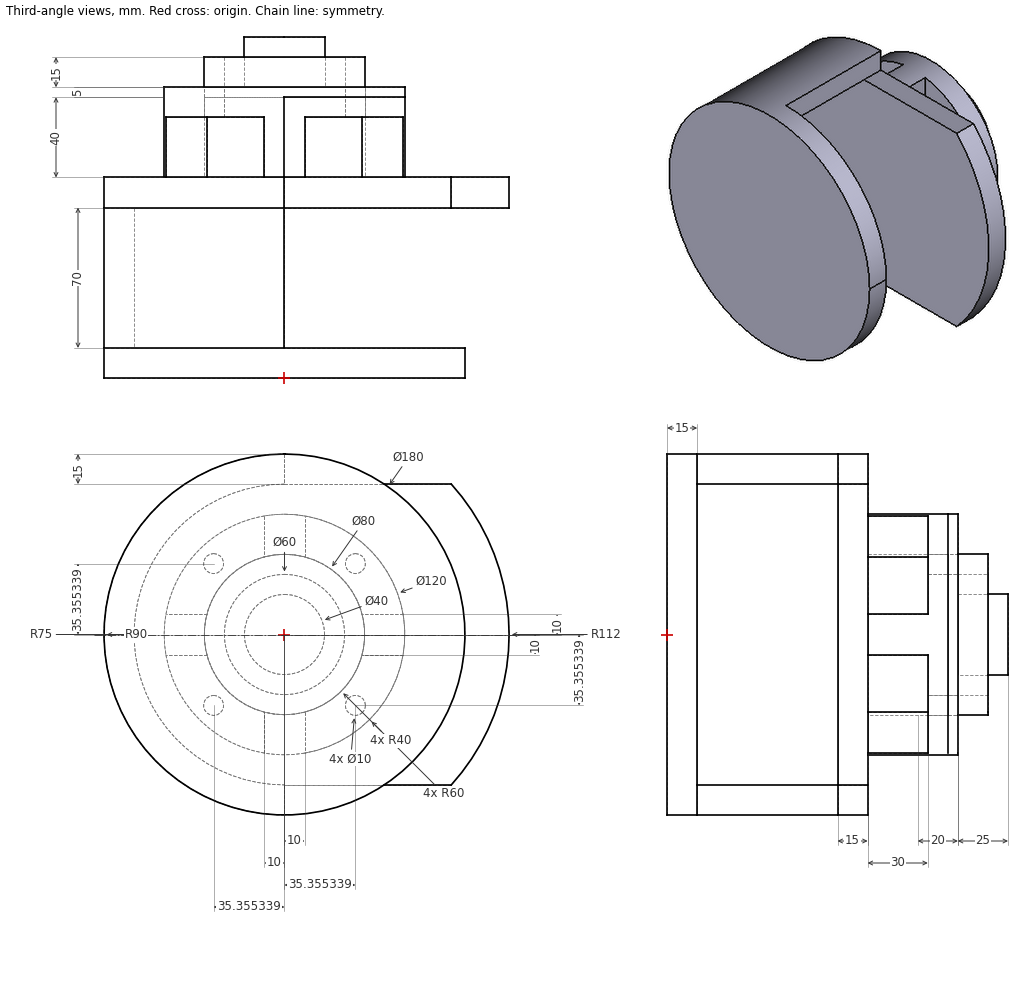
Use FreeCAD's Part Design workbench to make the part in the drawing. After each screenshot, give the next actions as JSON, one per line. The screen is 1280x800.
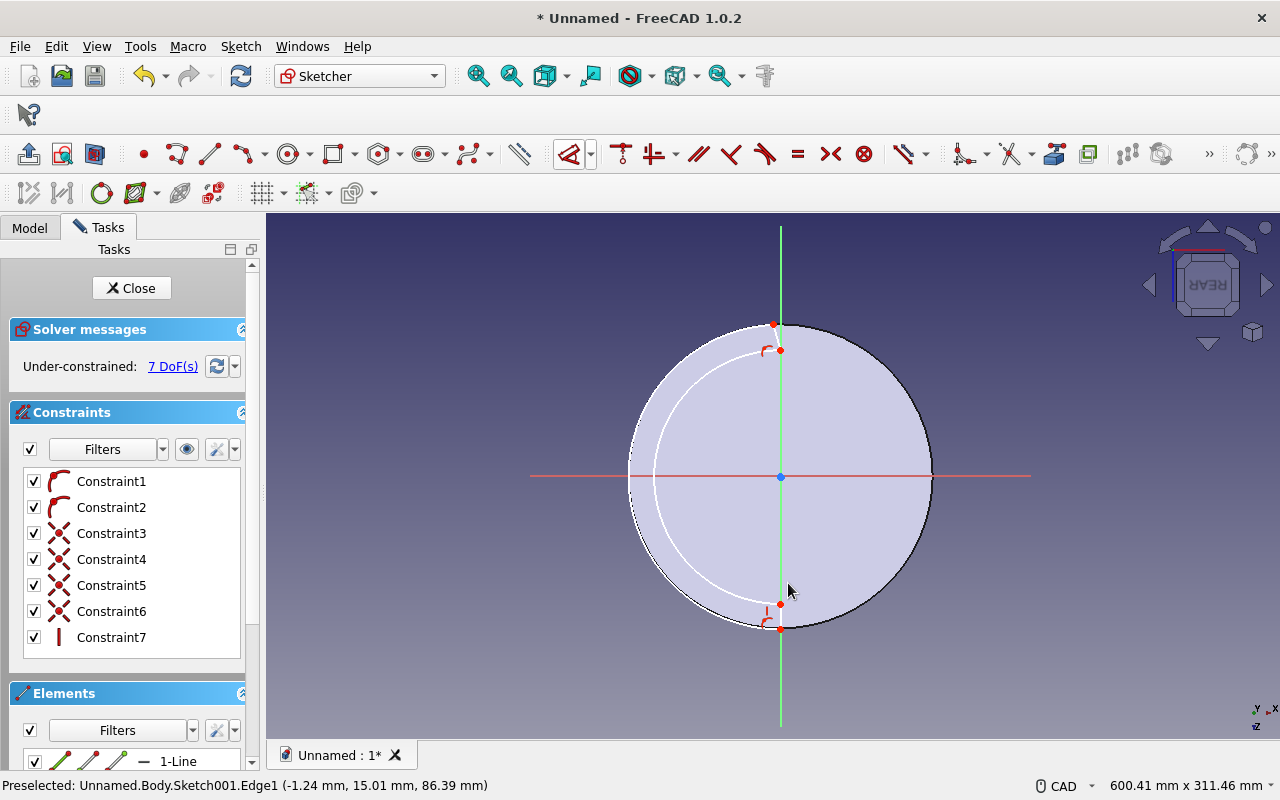
{"action": "scroll", "coordinate": [776, 332], "scroll_direction": "up", "scroll_amount": 5}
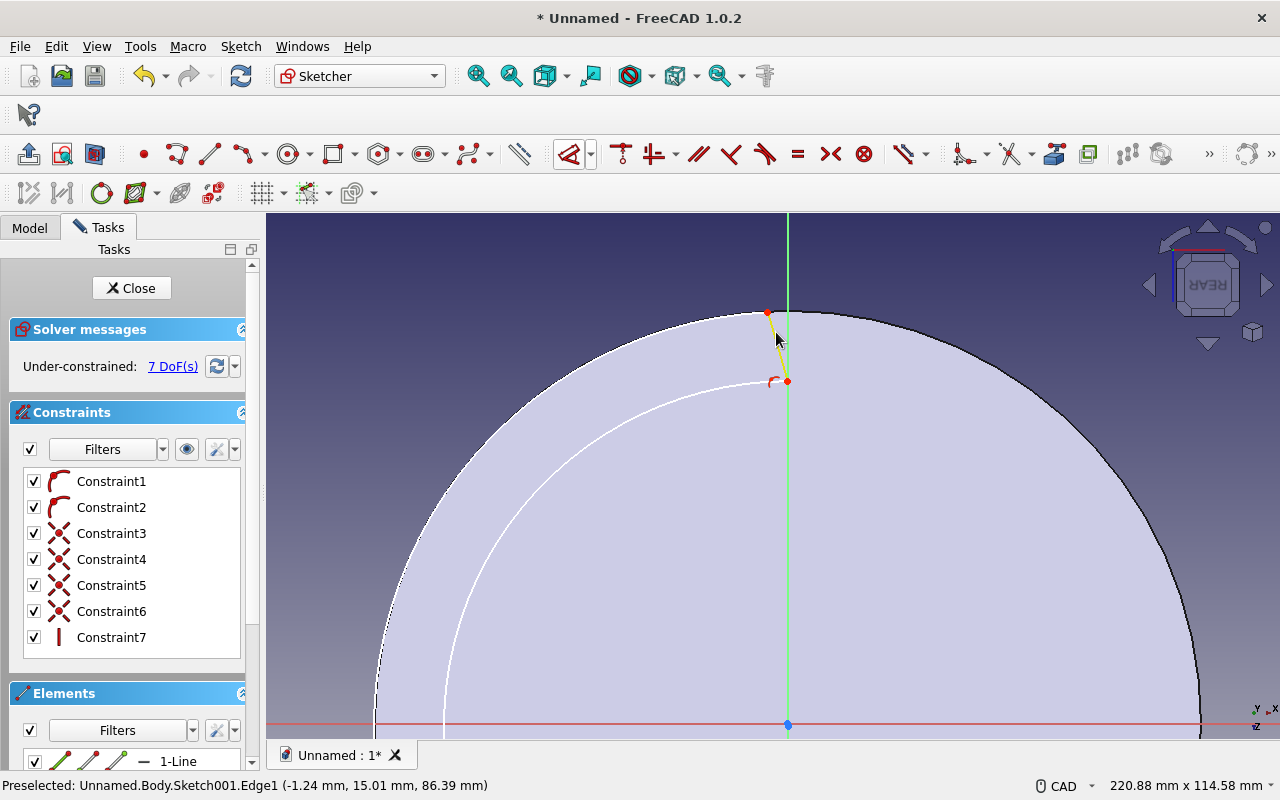
{"action": "left_click", "coordinate": [774, 333]}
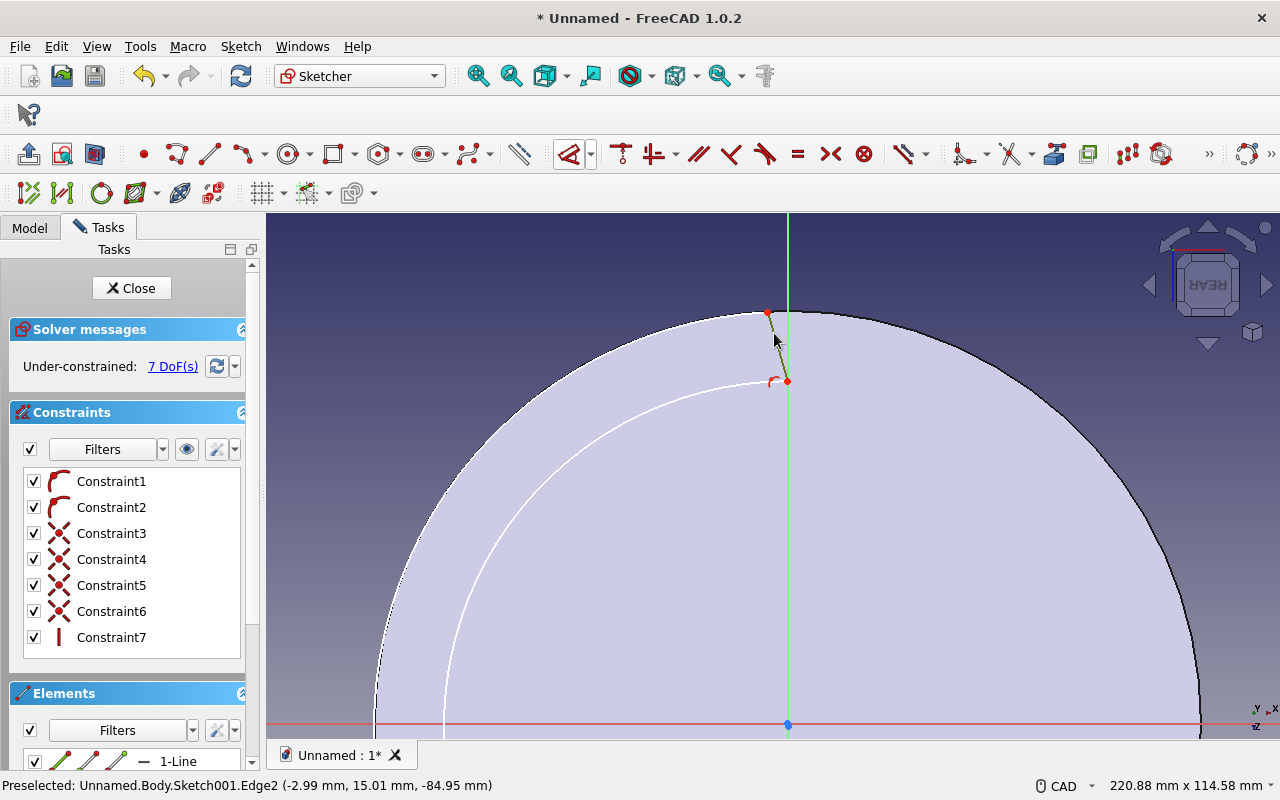
{"action": "key", "text": "v"}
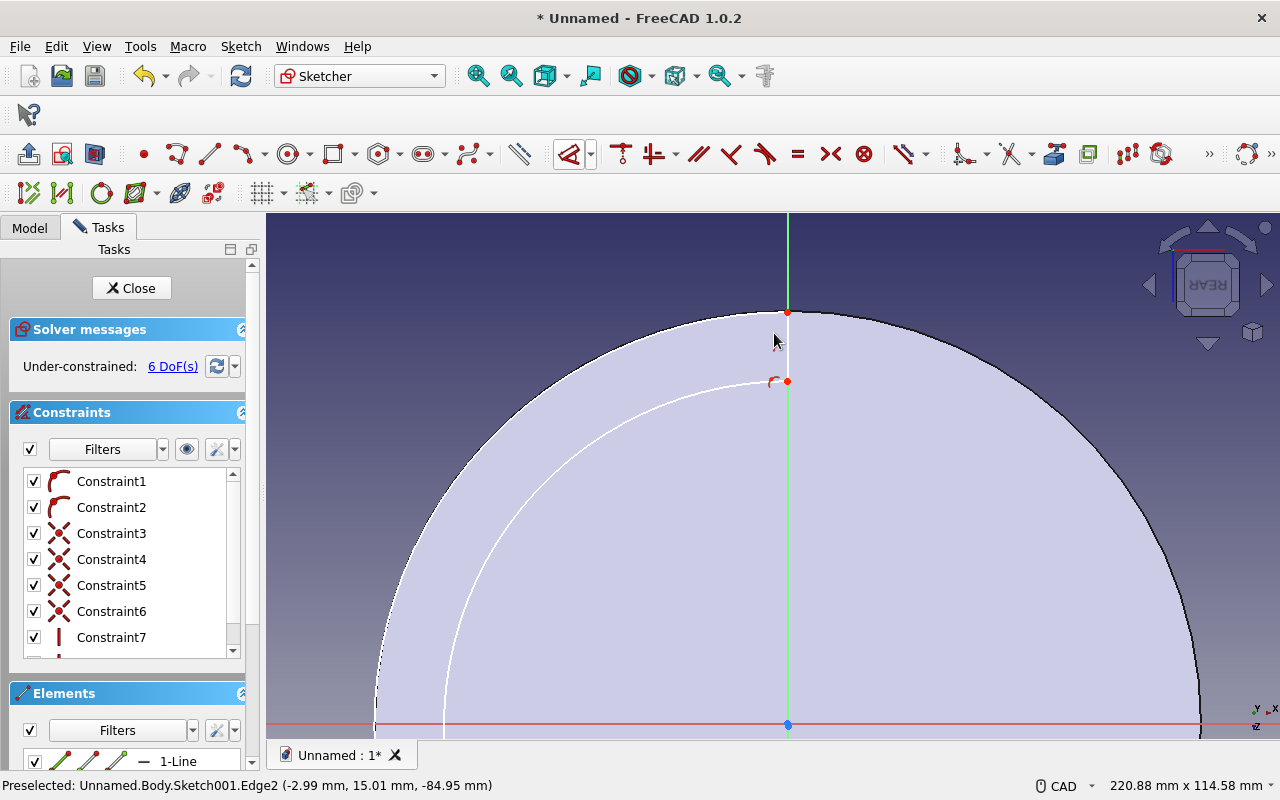
{"action": "left_click", "coordinate": [510, 524]}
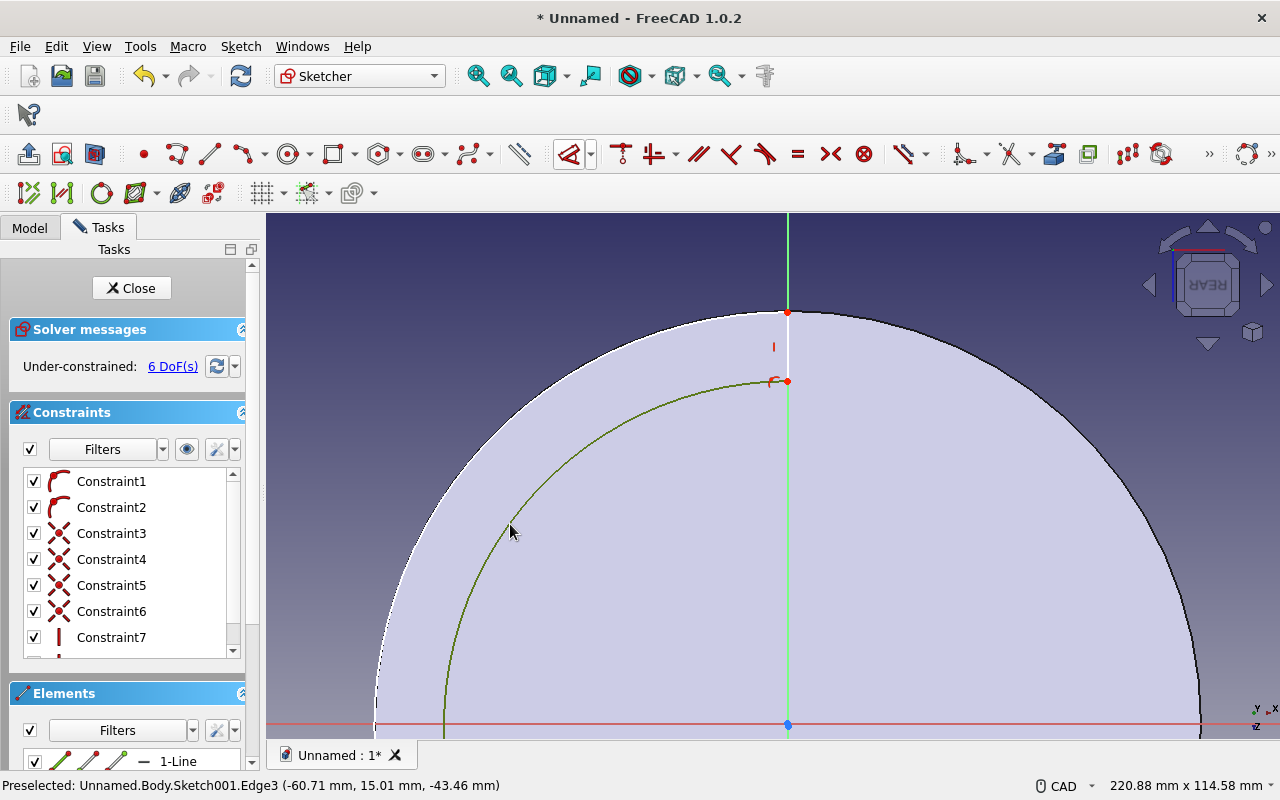
{"action": "left_click", "coordinate": [453, 483]}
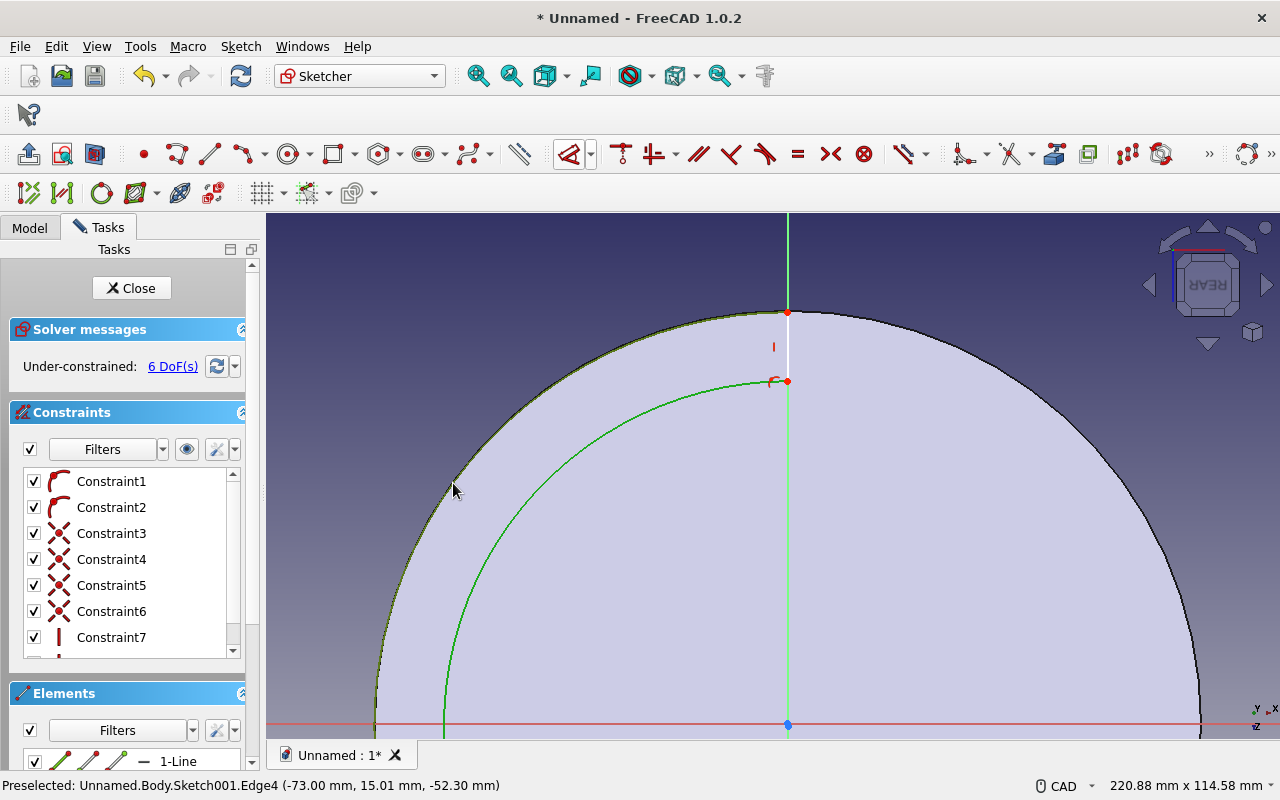
{"action": "left_click", "coordinate": [621, 154]}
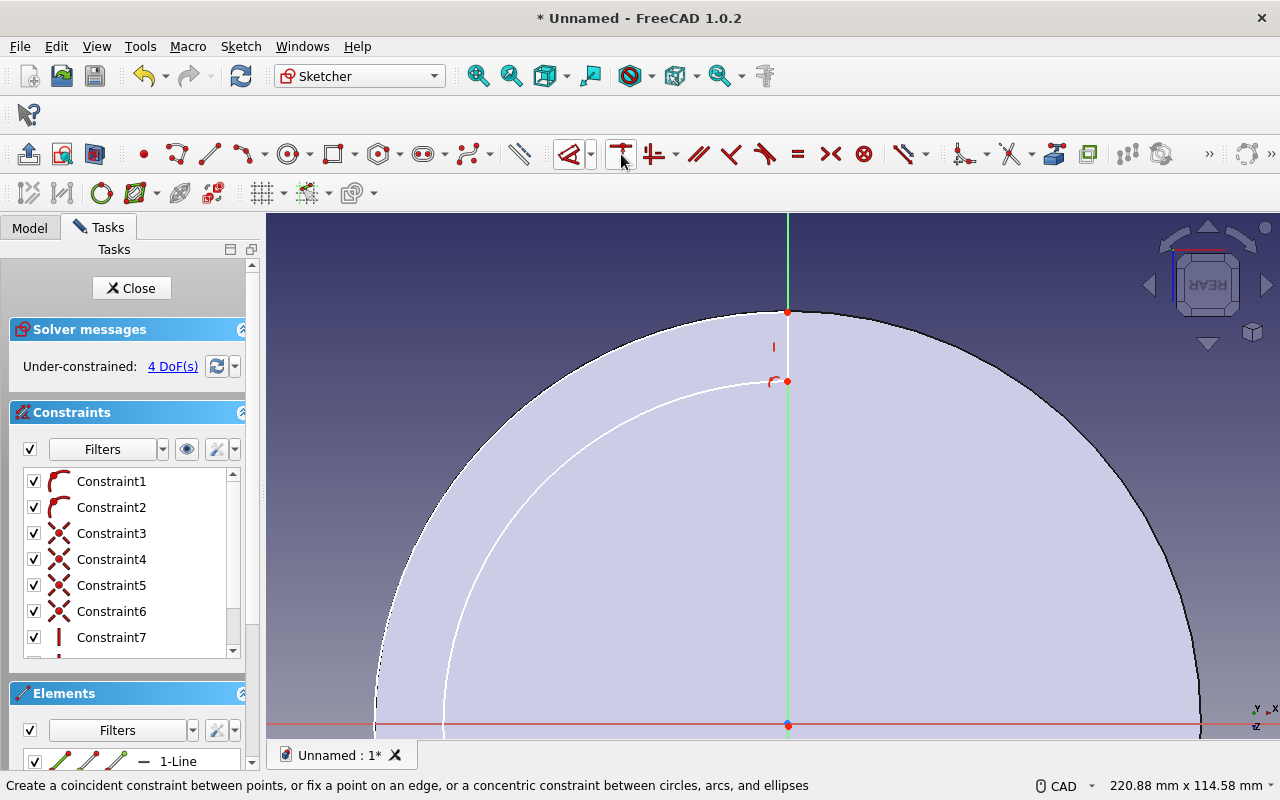
{"action": "scroll", "coordinate": [776, 332], "scroll_direction": "down", "scroll_amount": 5}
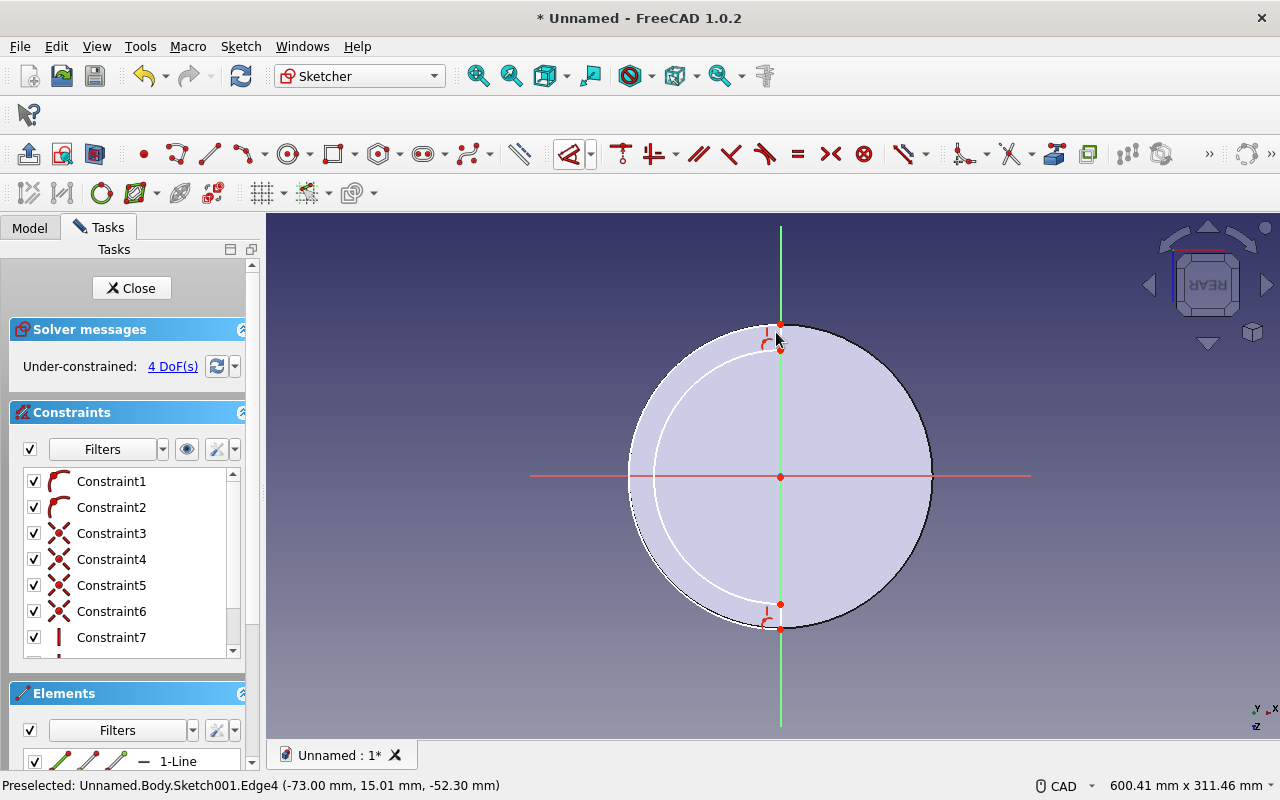
{"action": "left_click_drag", "start_coordinate": [771, 466], "coordinate": [791, 487]}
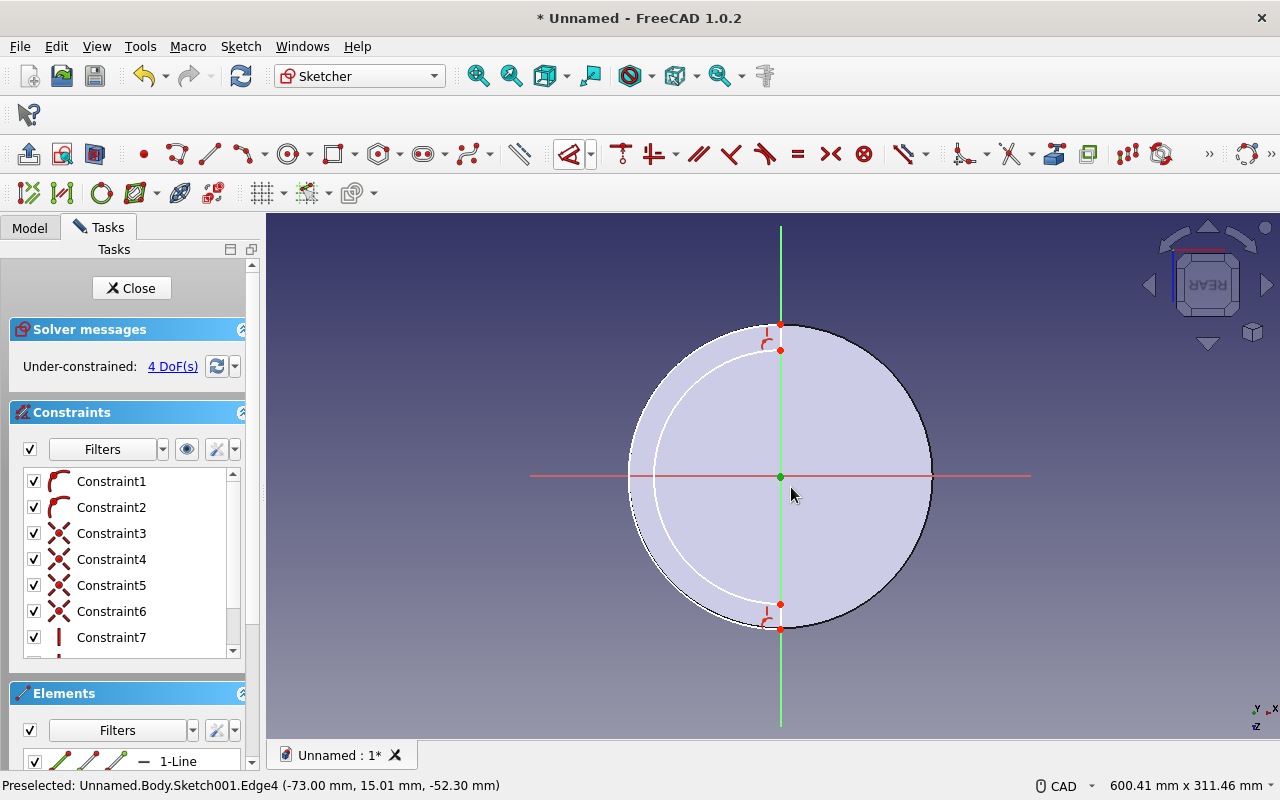
{"action": "left_click", "coordinate": [621, 154]}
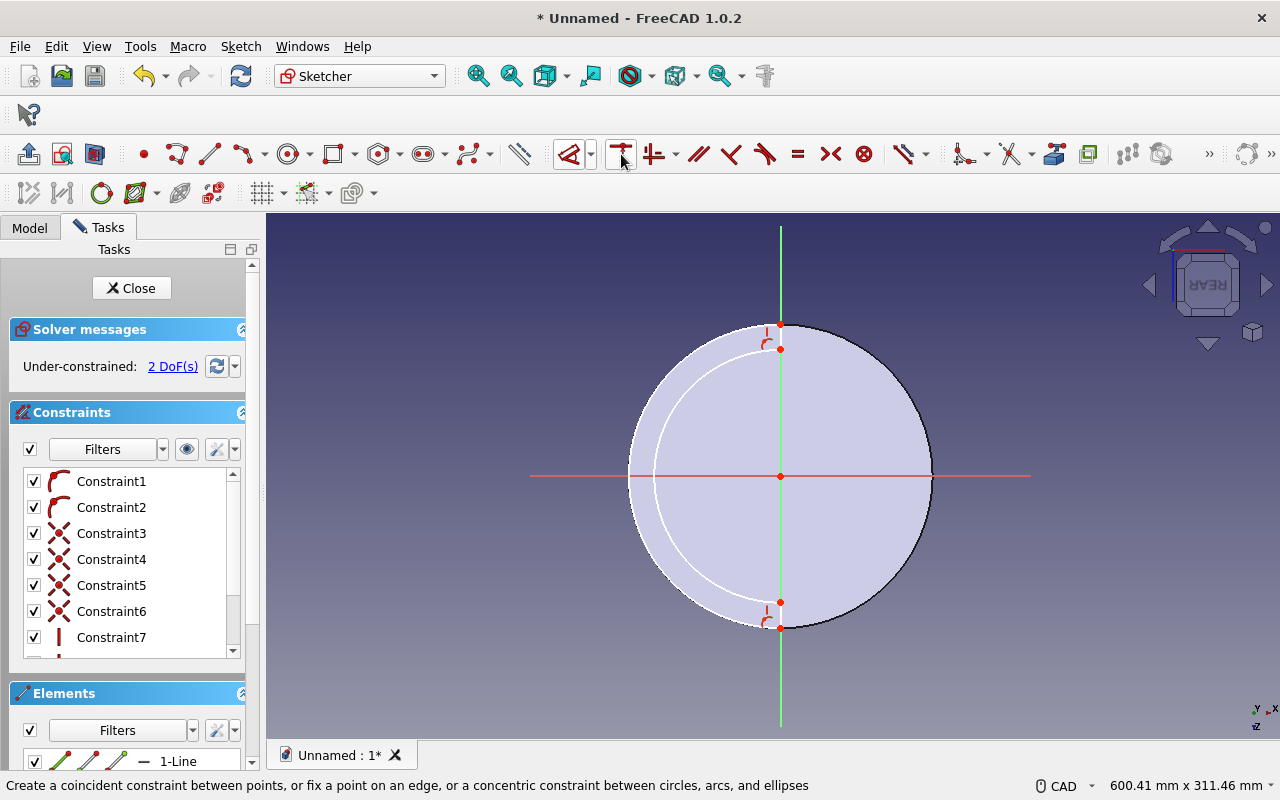
{"action": "left_click", "coordinate": [678, 402]}